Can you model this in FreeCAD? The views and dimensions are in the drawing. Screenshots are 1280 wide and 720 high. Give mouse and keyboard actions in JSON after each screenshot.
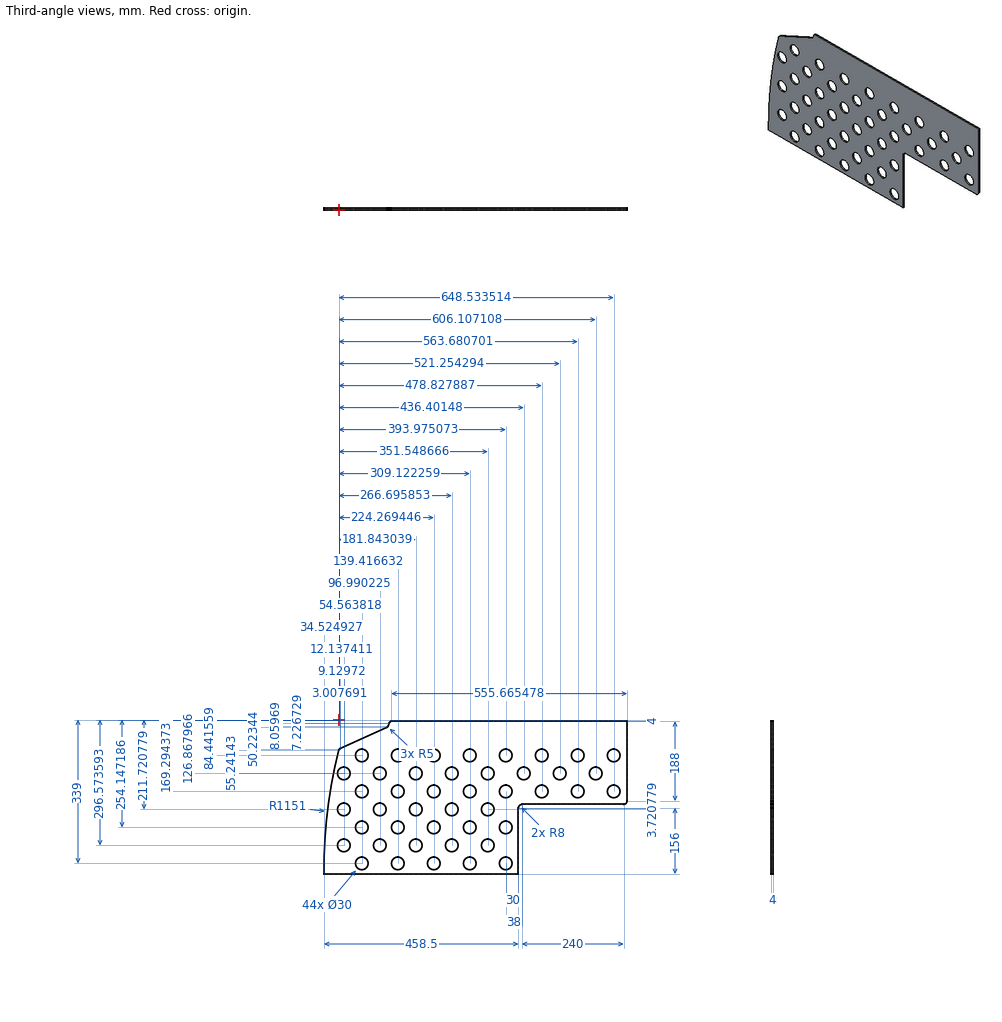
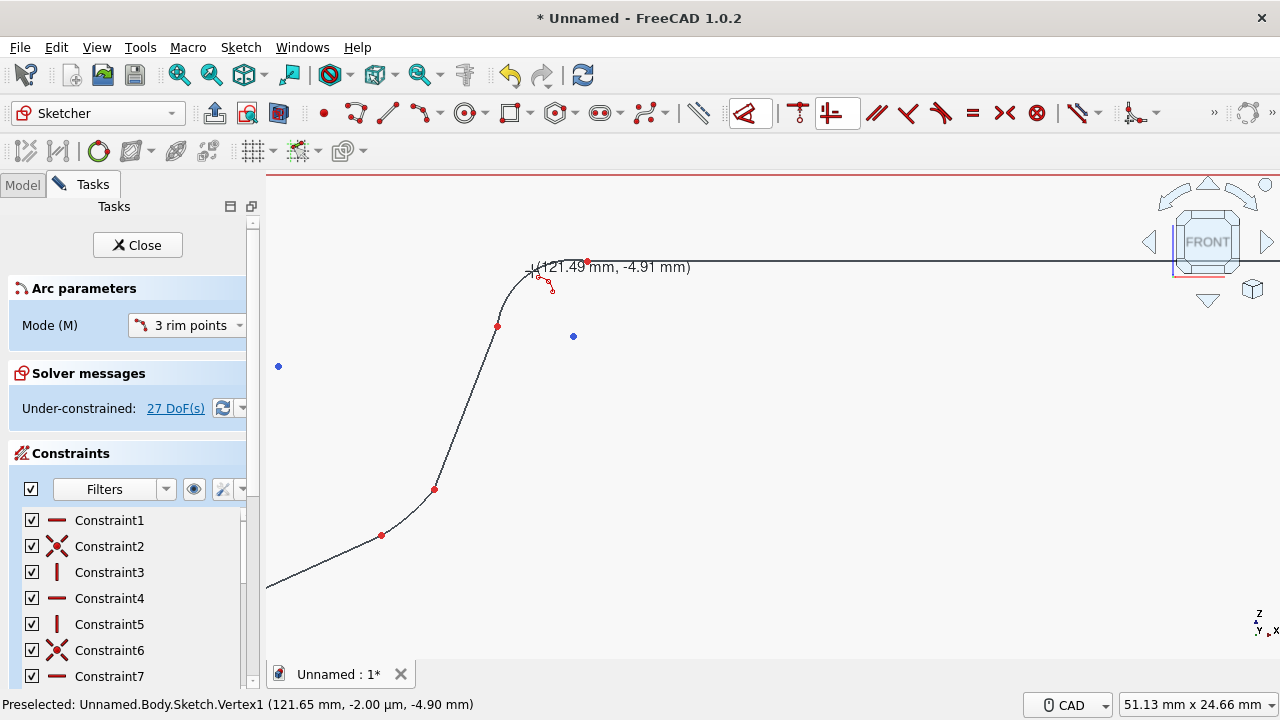
{"action": "key", "text": "g c"}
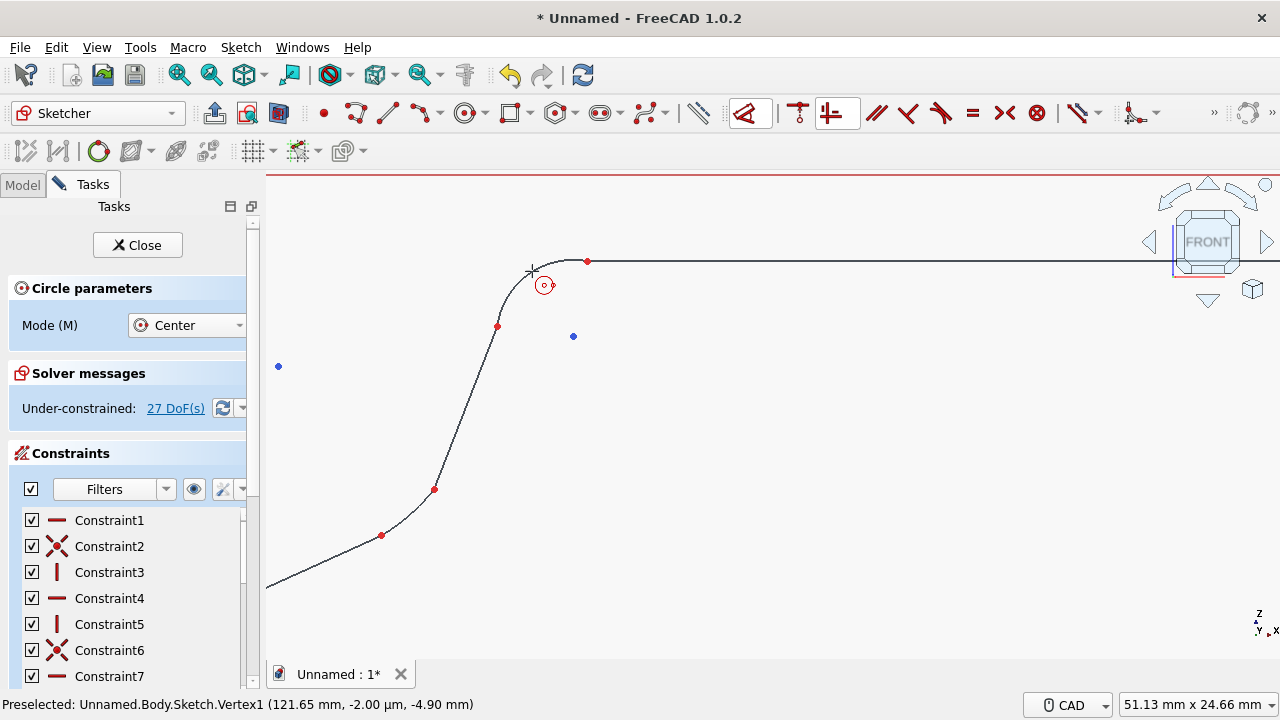
{"action": "scroll", "coordinate": [504, 238], "scroll_direction": "down", "scroll_amount": 15}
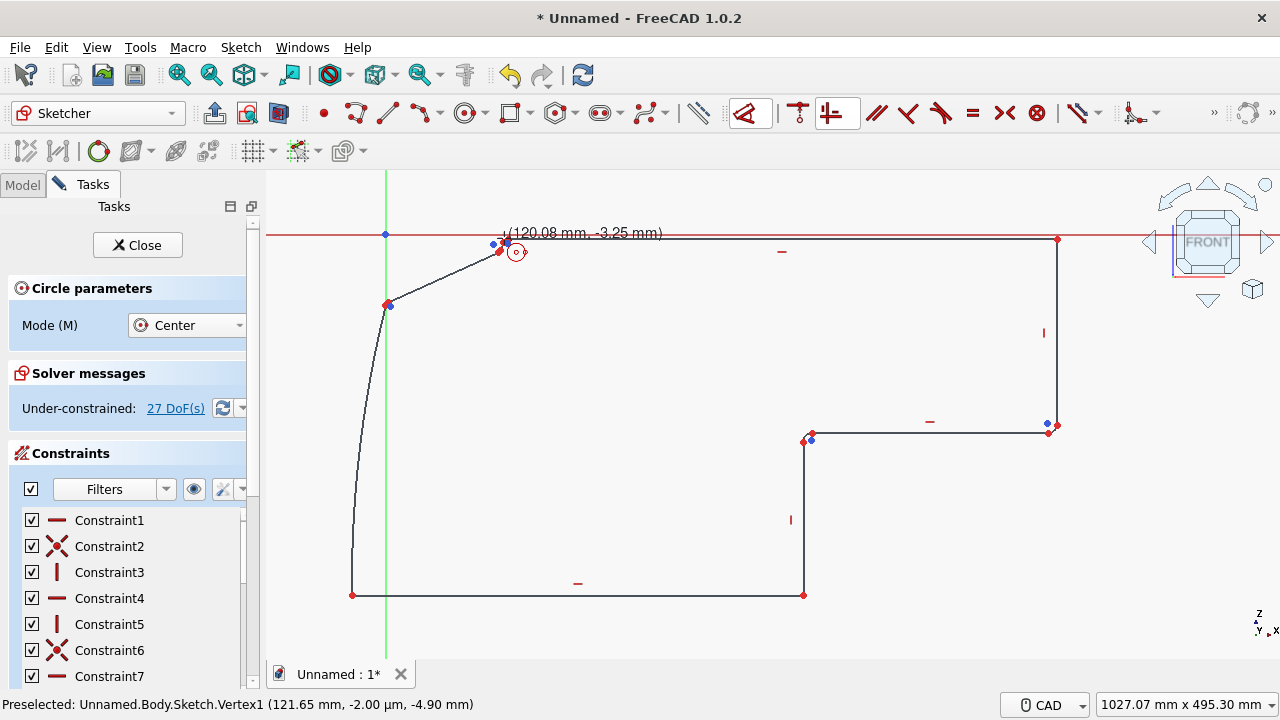
{"action": "scroll", "coordinate": [440, 570], "scroll_direction": "up", "scroll_amount": 3}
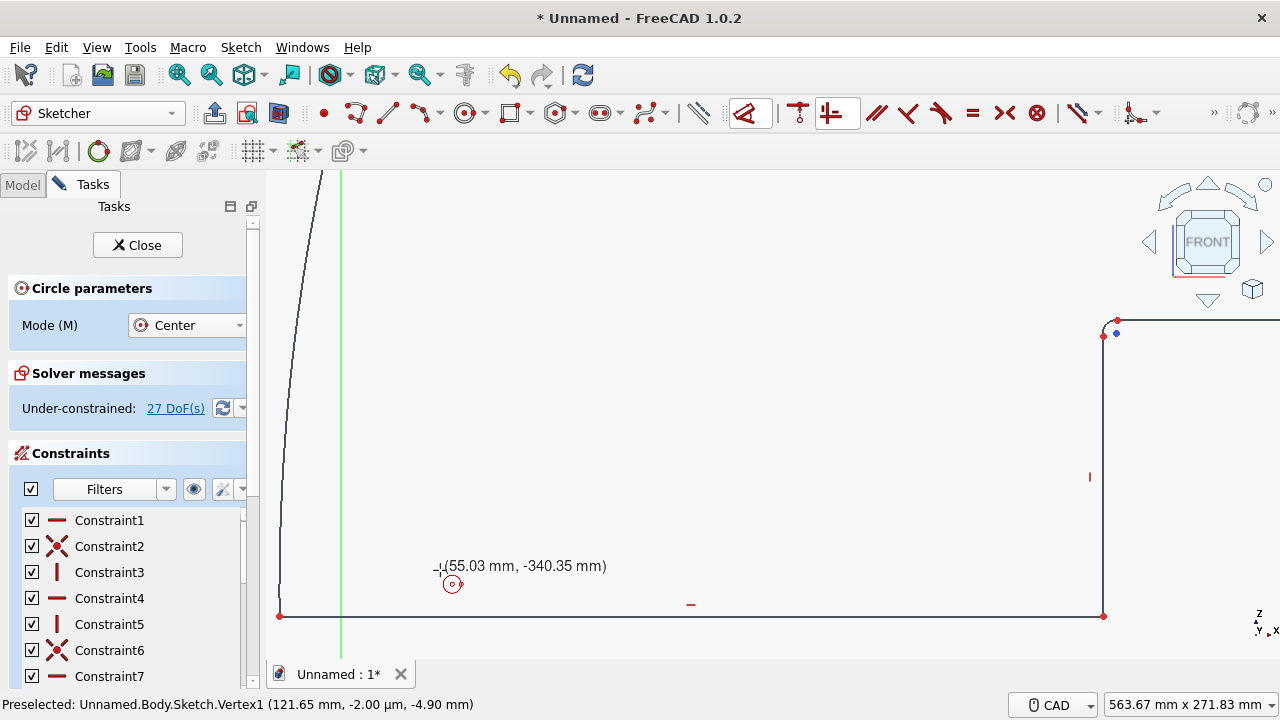
{"action": "left_click", "coordinate": [439, 569]}
{"action": "left_click", "coordinate": [458, 550]}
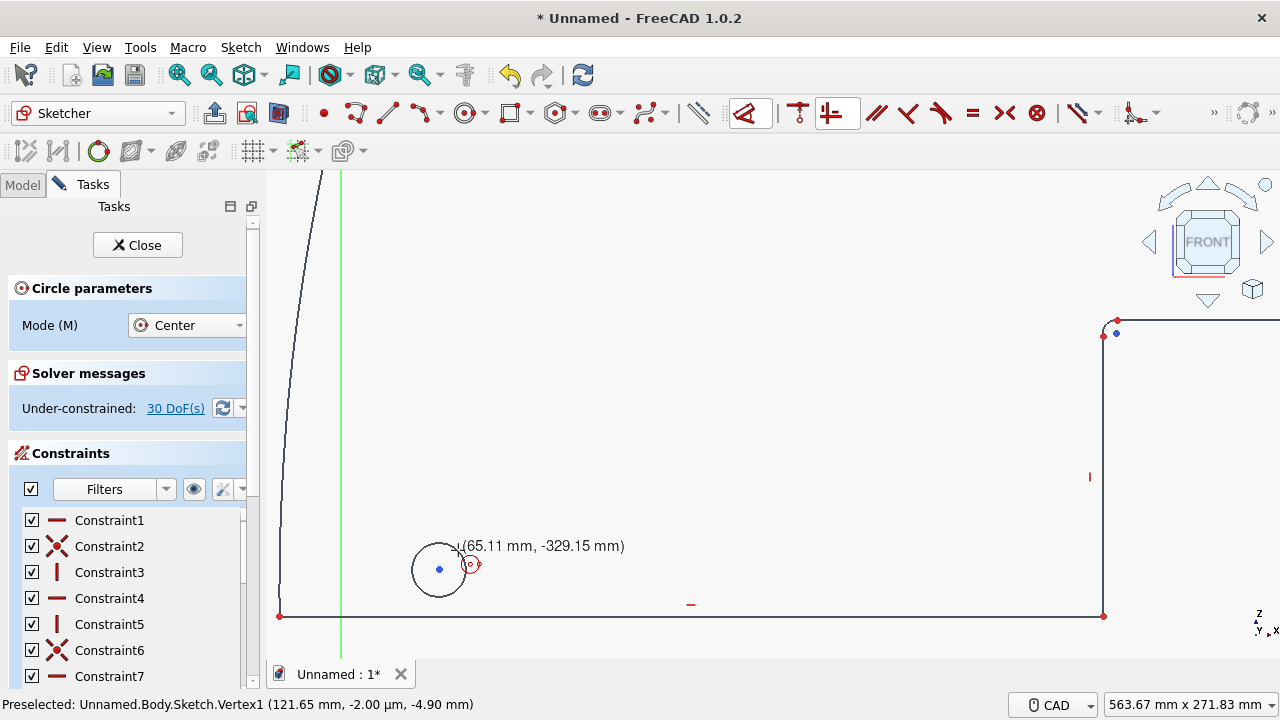
{"action": "left_click", "coordinate": [592, 569]}
{"action": "left_click", "coordinate": [611, 550]}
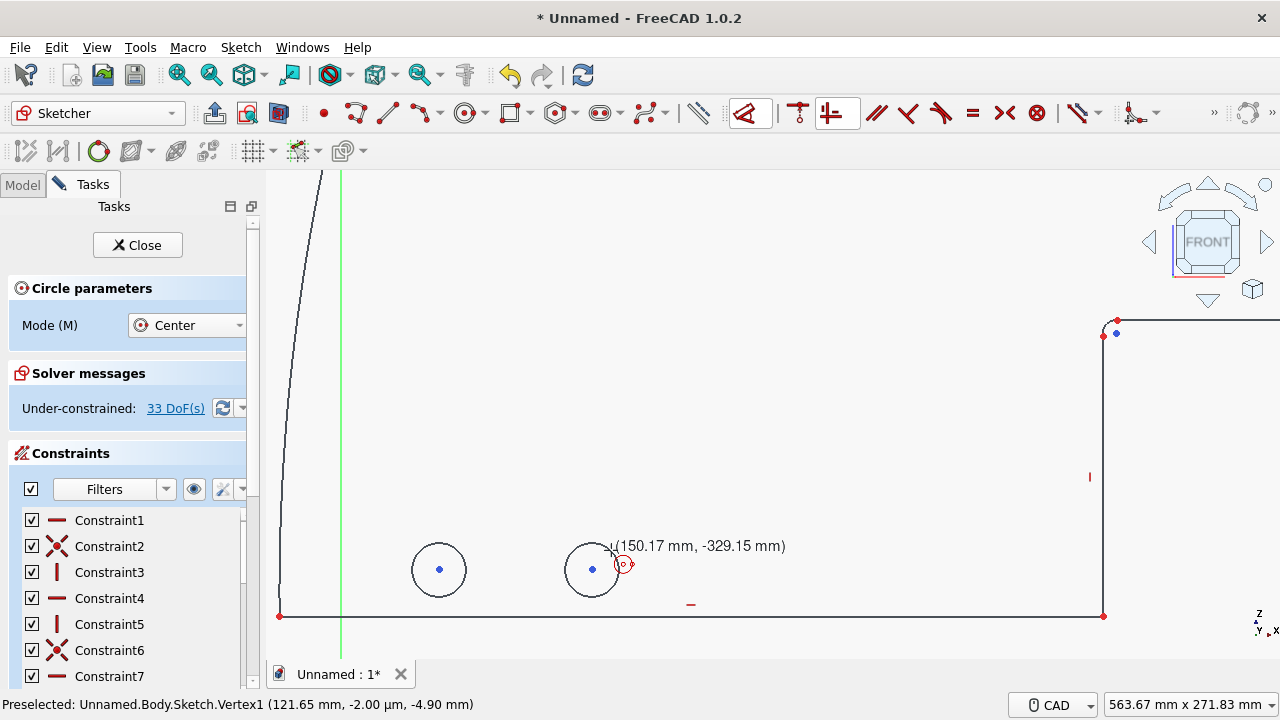
{"action": "left_click", "coordinate": [363, 492]}
{"action": "left_click", "coordinate": [382, 473]}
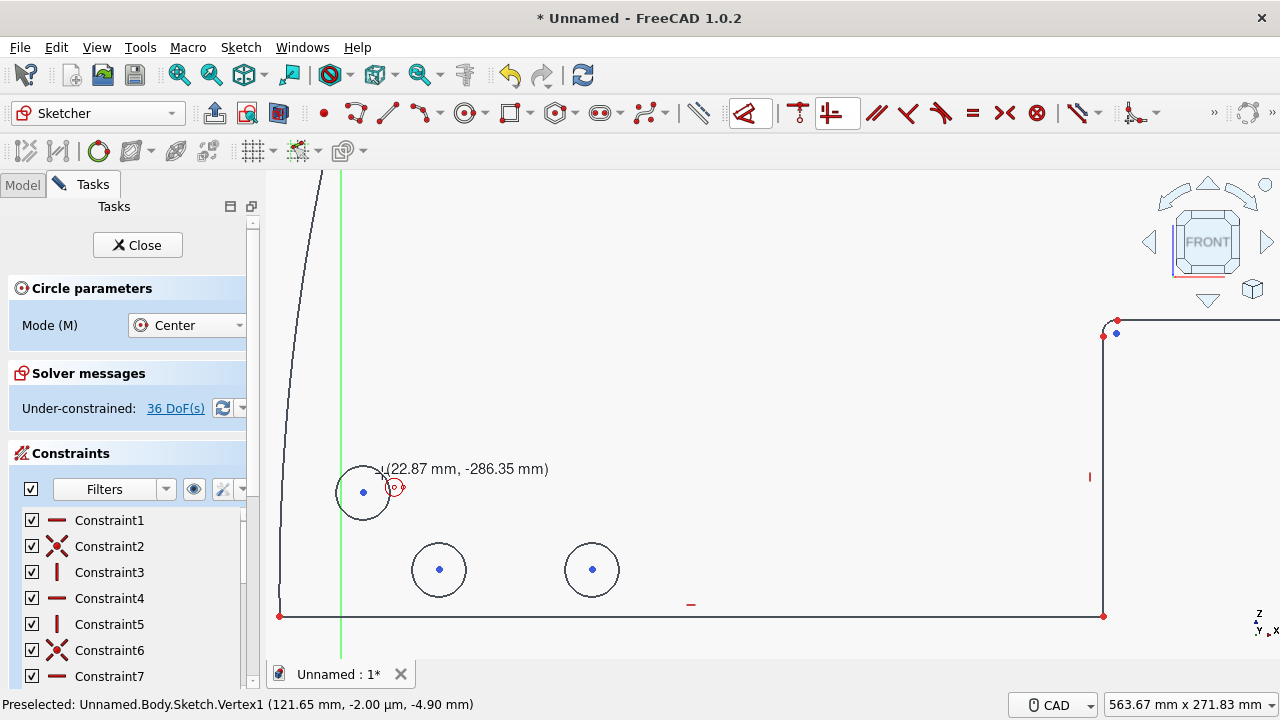
{"action": "left_click", "coordinate": [515, 492]}
{"action": "left_click", "coordinate": [534, 473]}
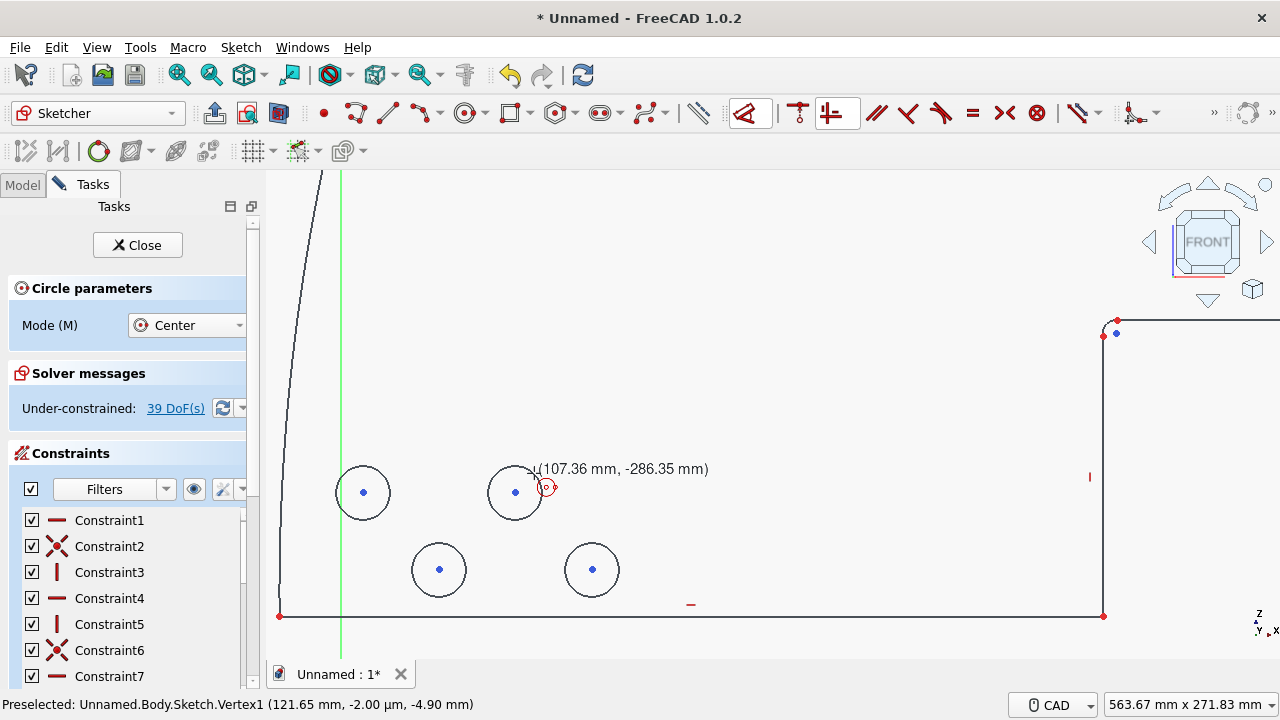
{"action": "left_click", "coordinate": [744, 569]}
{"action": "left_click", "coordinate": [763, 550]}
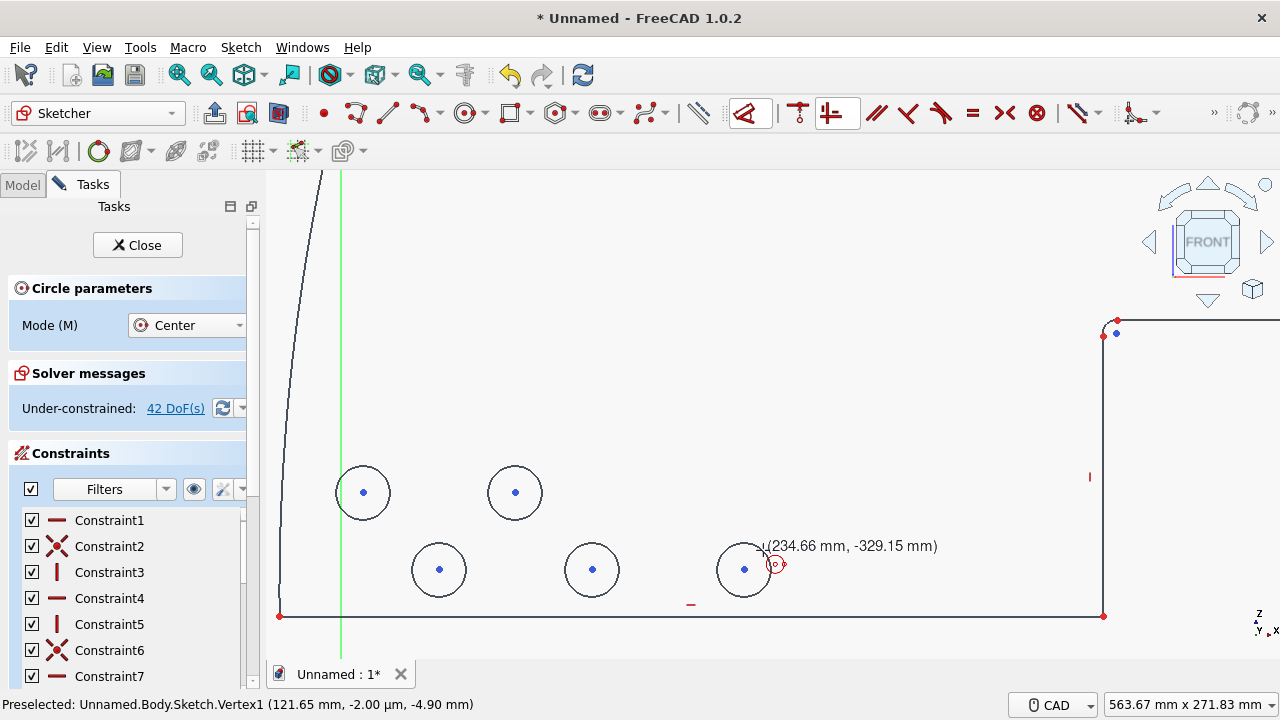
{"action": "left_click", "coordinate": [897, 569]}
{"action": "left_click", "coordinate": [916, 550]}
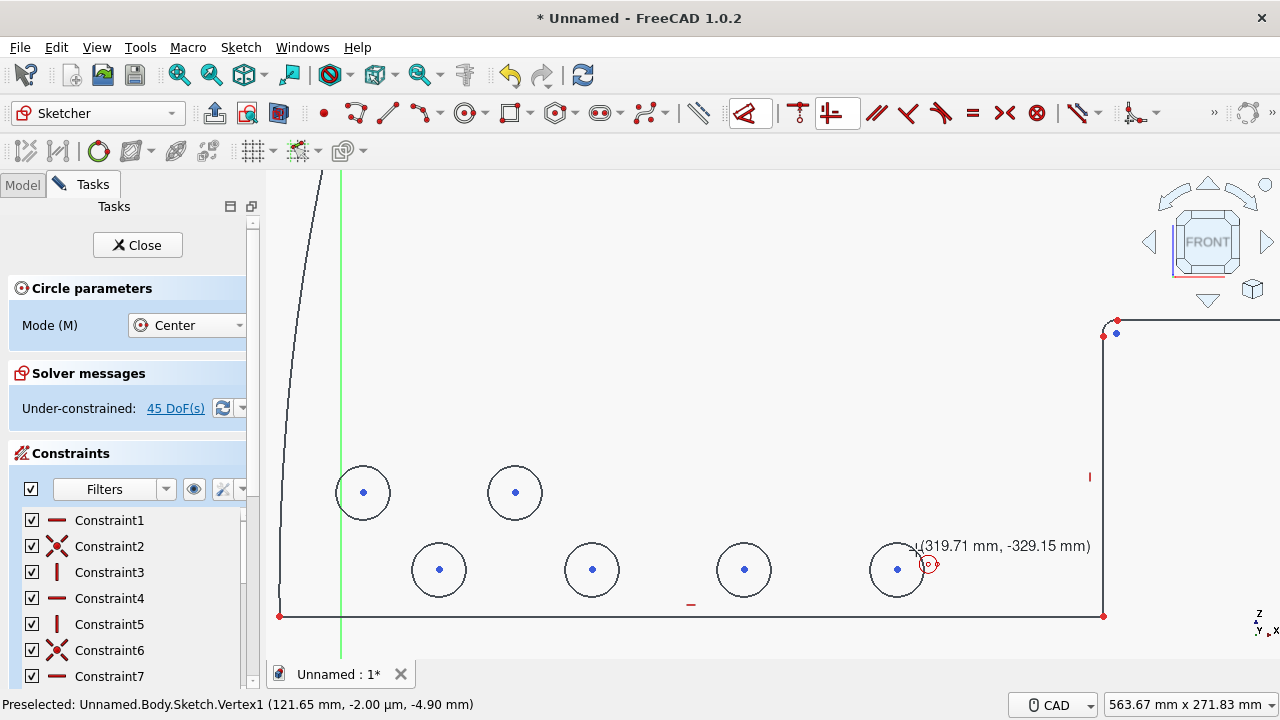
{"action": "left_click", "coordinate": [668, 492]}
{"action": "left_click", "coordinate": [687, 473]}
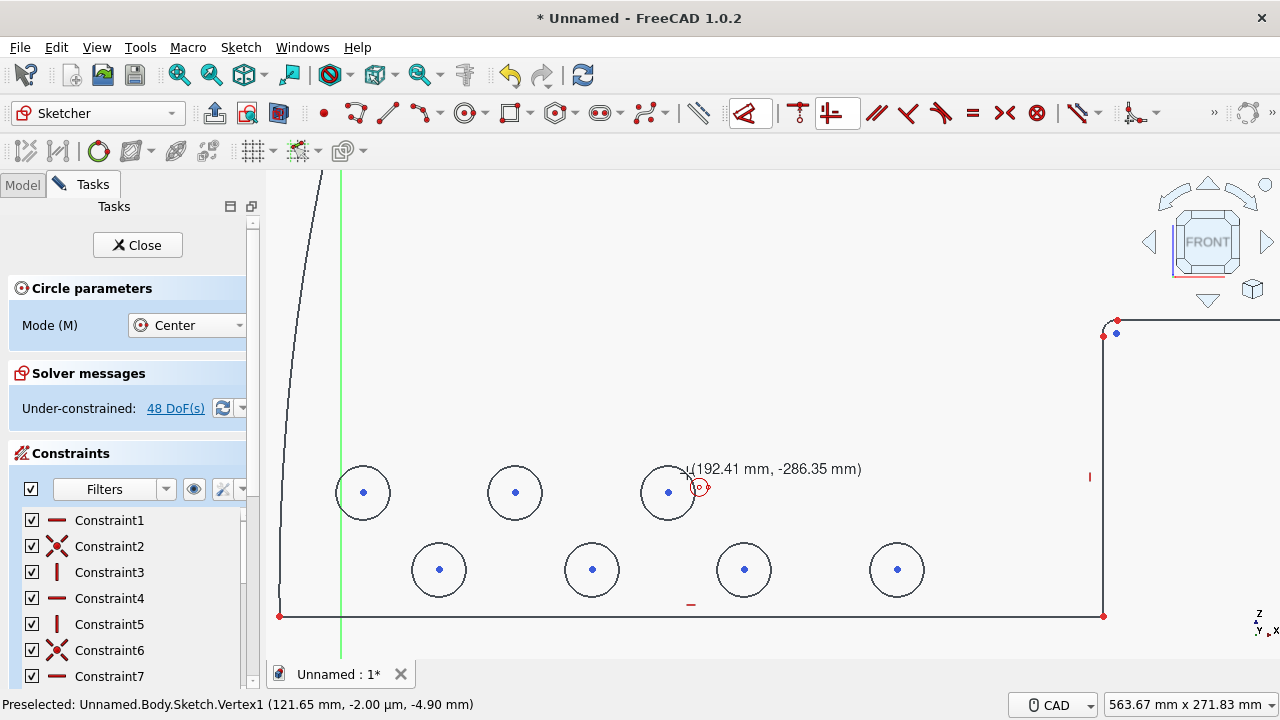
{"action": "left_click", "coordinate": [821, 492]}
{"action": "left_click", "coordinate": [840, 473]}